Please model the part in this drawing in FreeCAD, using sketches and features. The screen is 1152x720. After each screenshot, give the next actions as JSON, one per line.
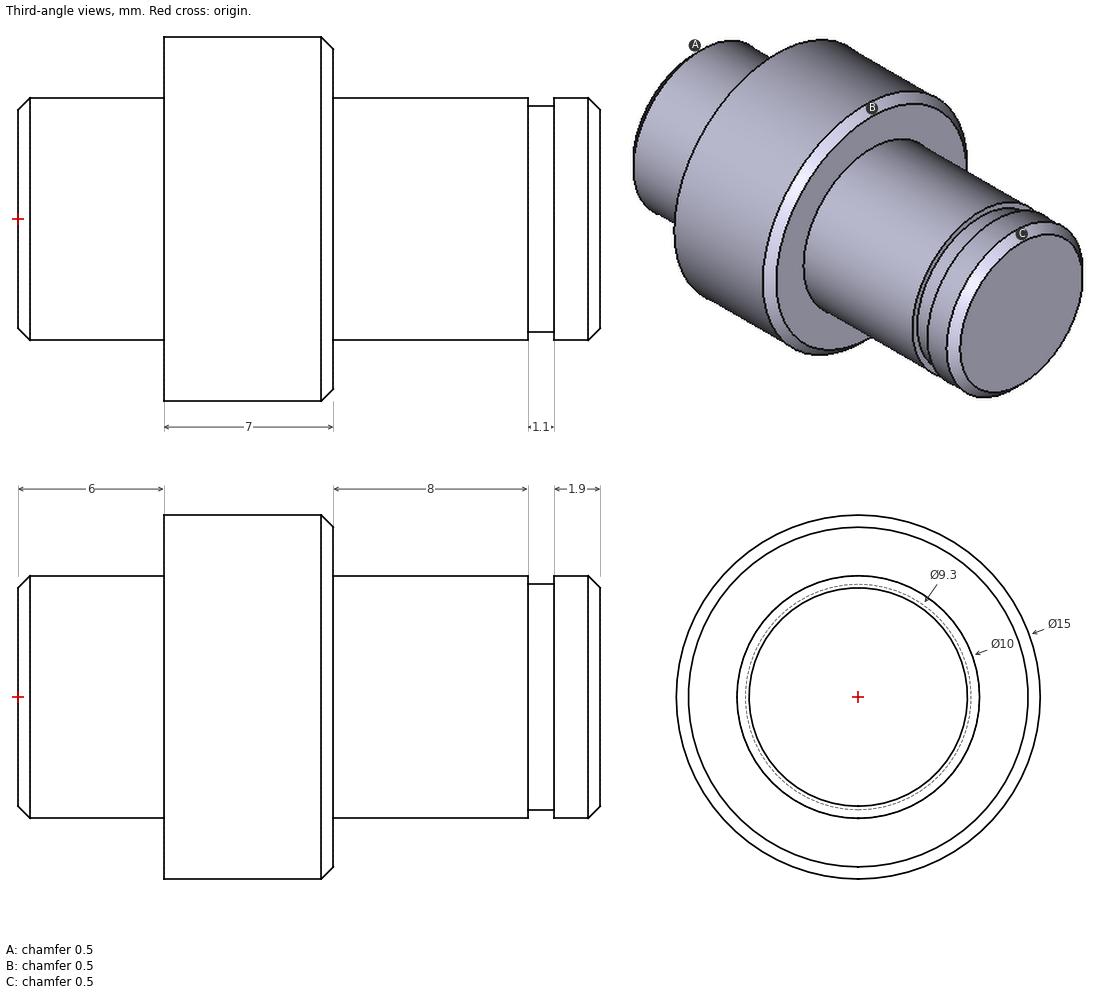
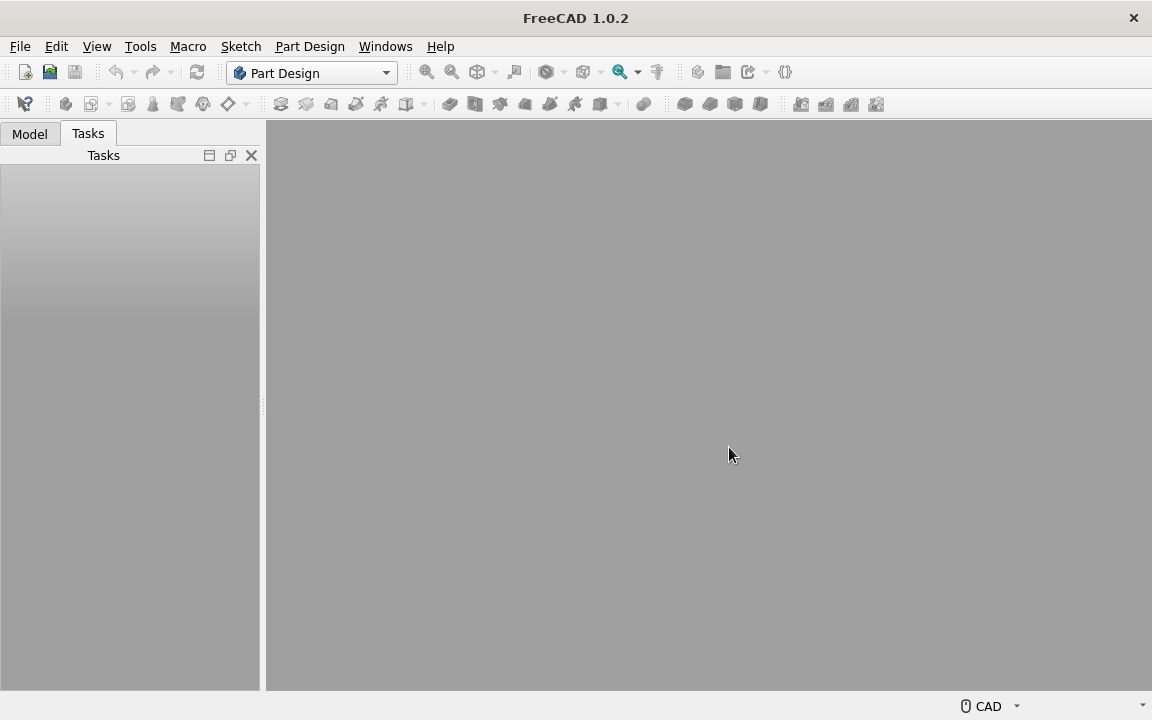
{"action": "left_click", "coordinate": [25, 72]}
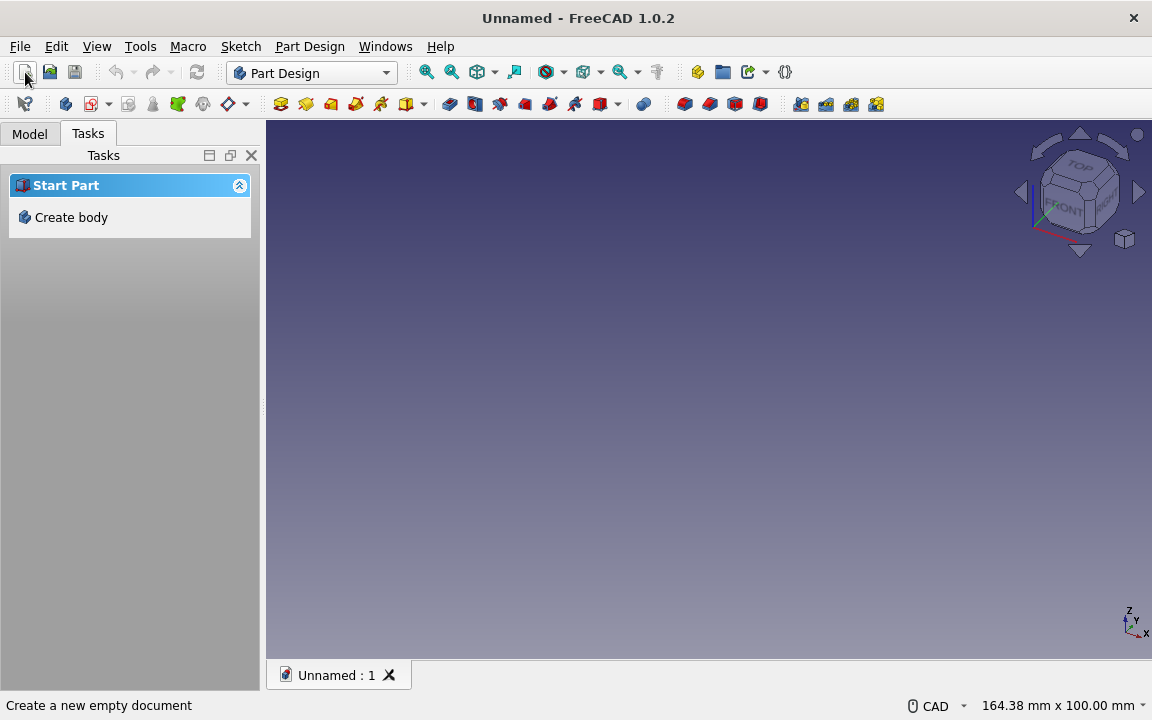
{"action": "left_click", "coordinate": [90, 104]}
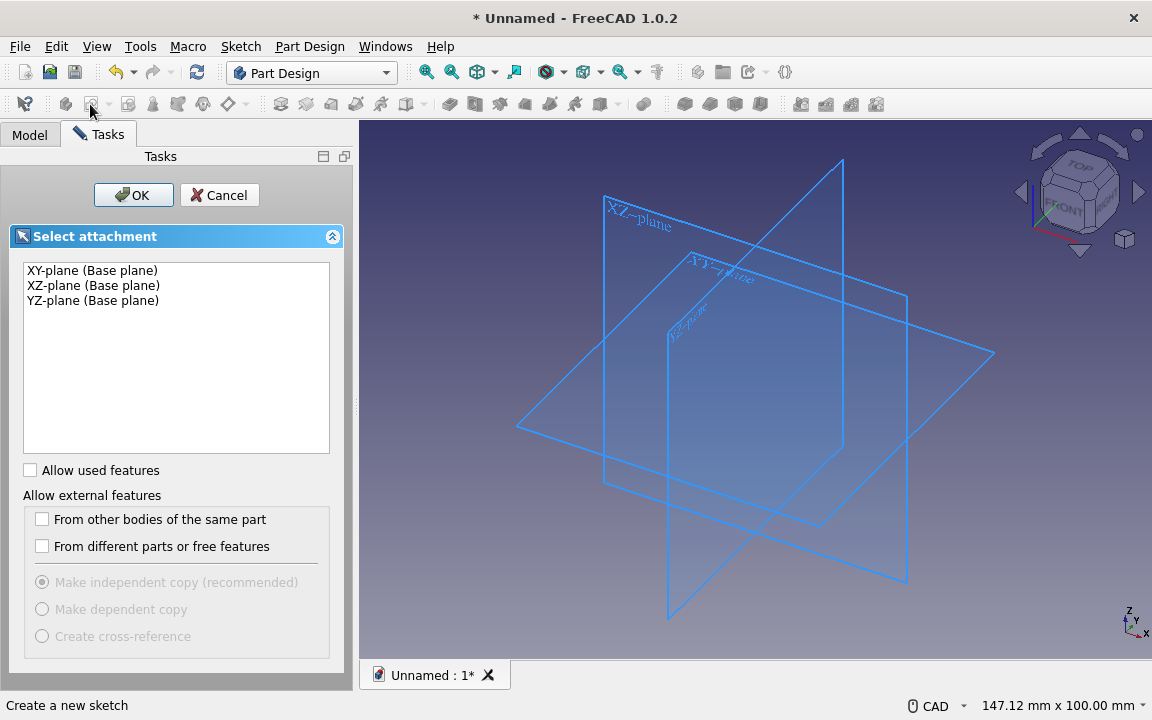
{"action": "left_click", "coordinate": [84, 300]}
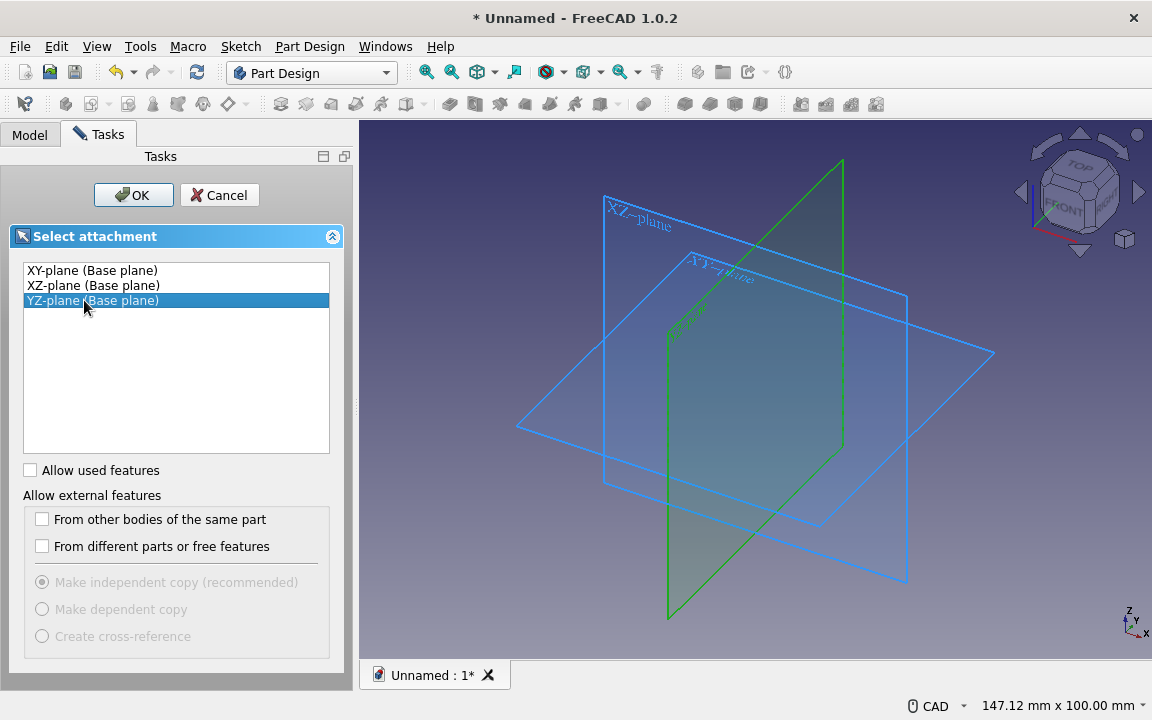
{"action": "left_click", "coordinate": [134, 195]}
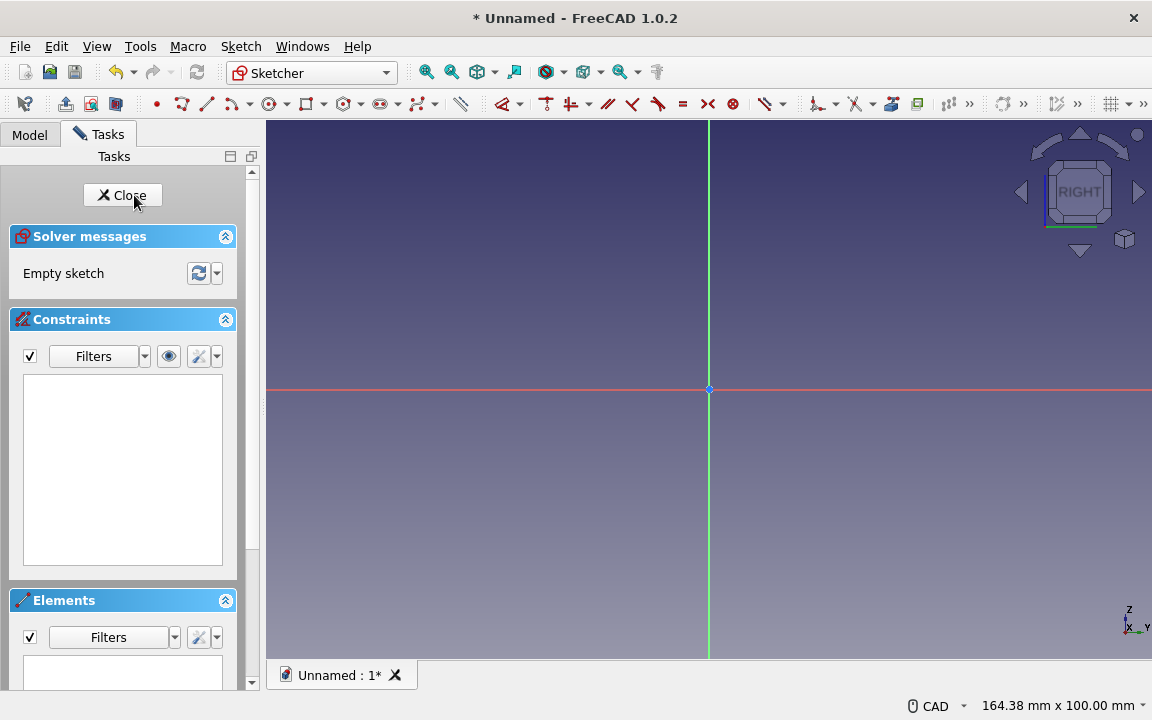
{"action": "scroll", "coordinate": [723, 390], "scroll_direction": "up", "scroll_amount": 9}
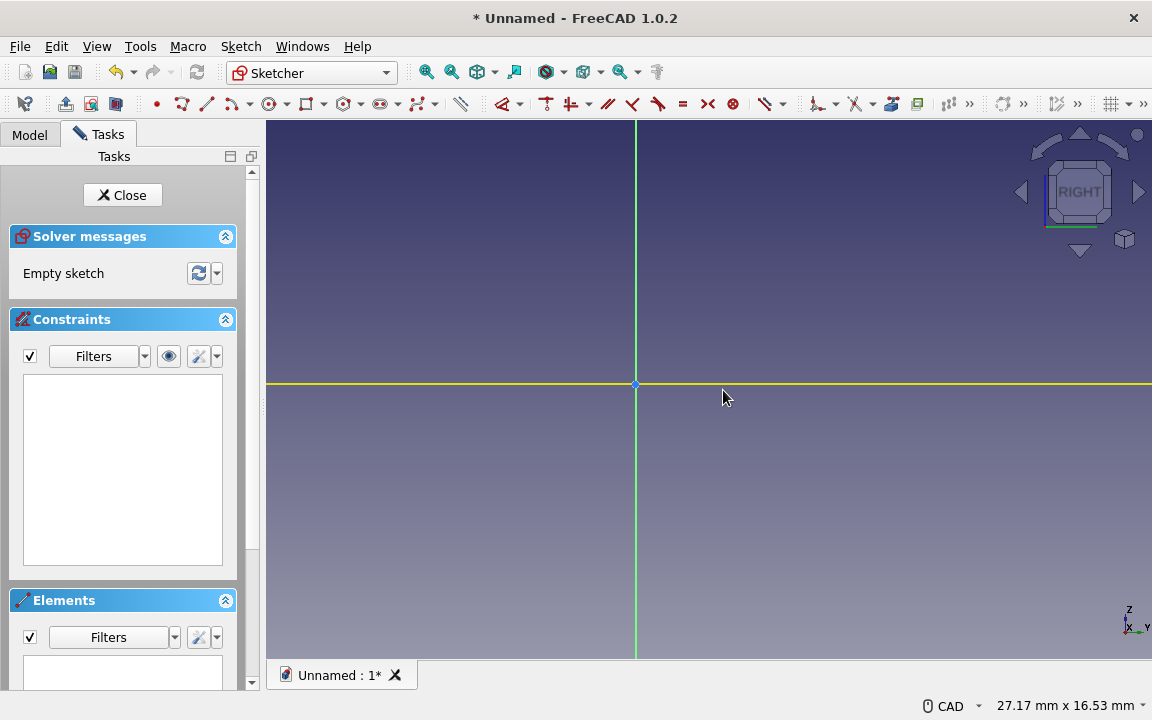
{"action": "key", "text": "g c"}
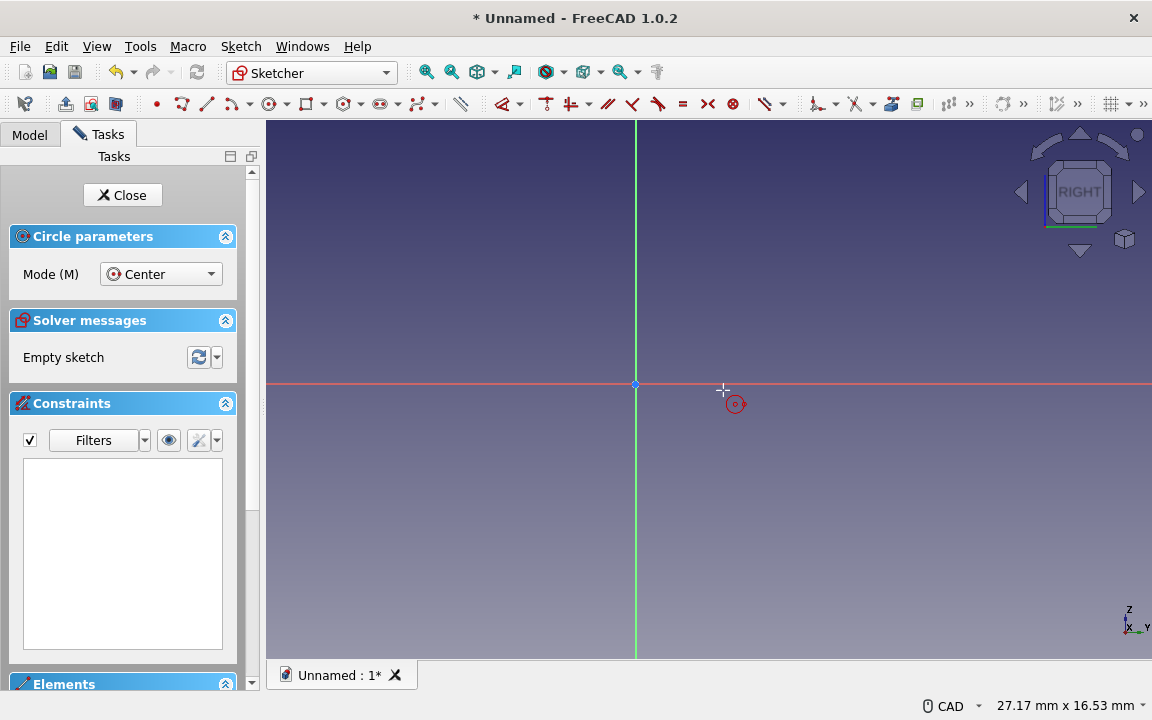
{"action": "left_click", "coordinate": [636, 384]}
{"action": "mouse_move", "coordinate": [751, 269]}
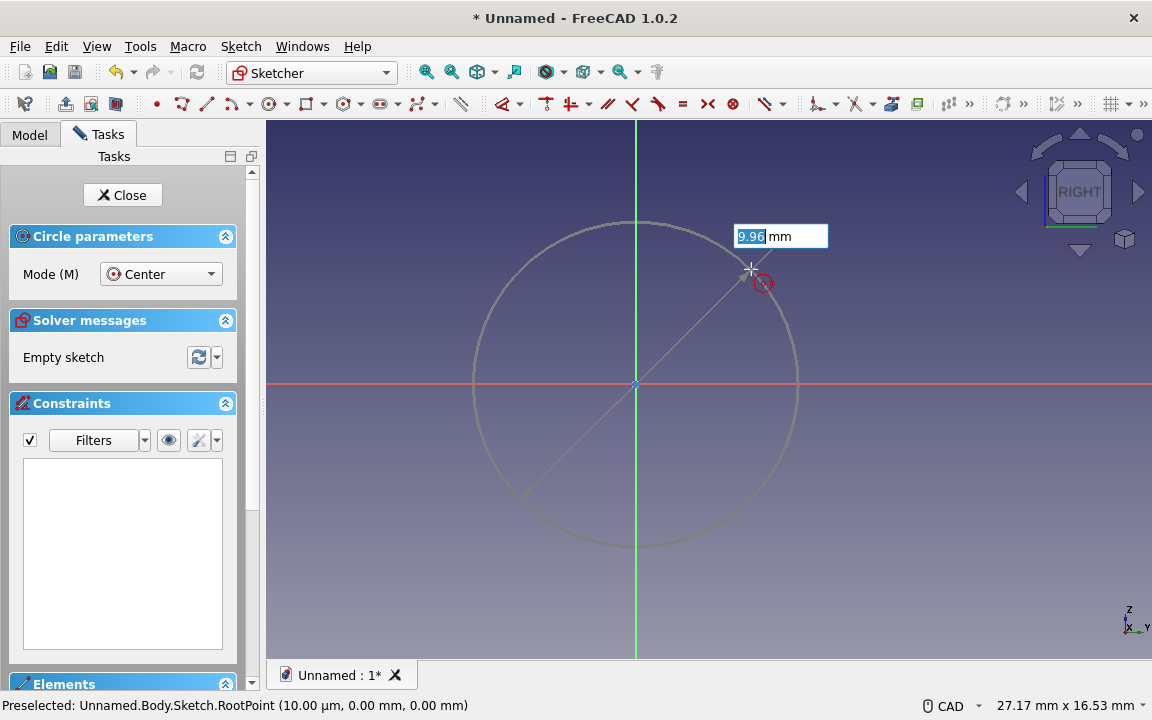
{"action": "type", "text": "10"}
{"action": "key", "text": "Return"}
{"action": "key", "text": "Escape"}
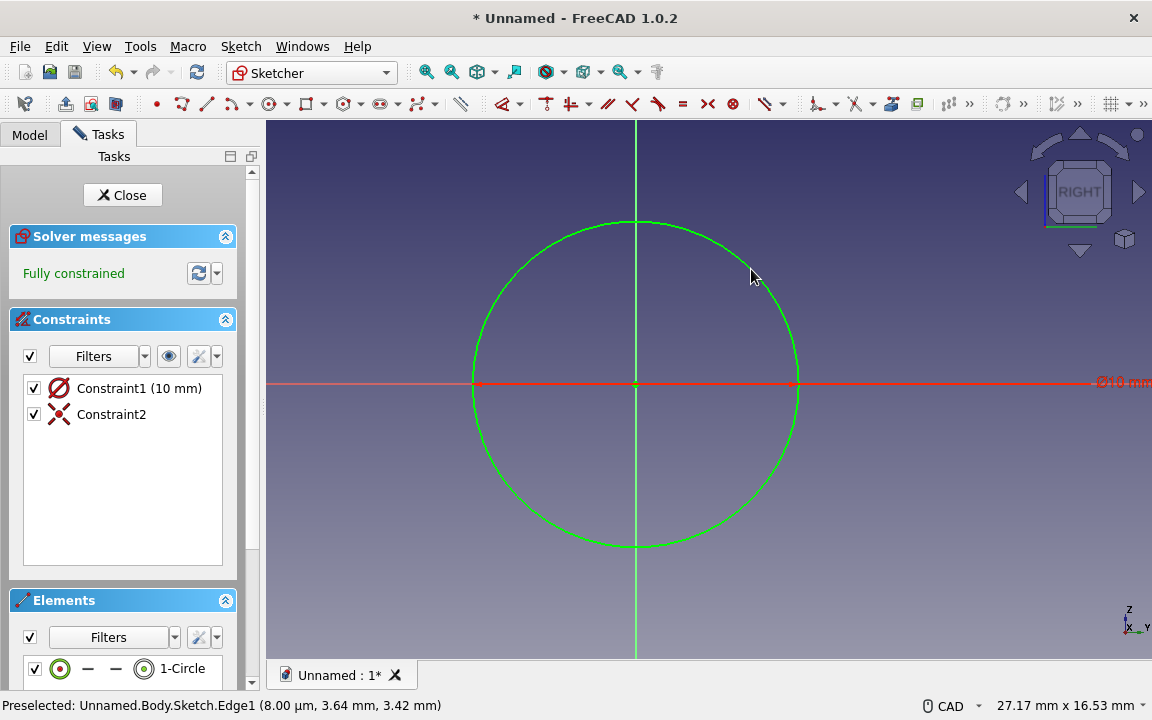
{"action": "left_click", "coordinate": [123, 195]}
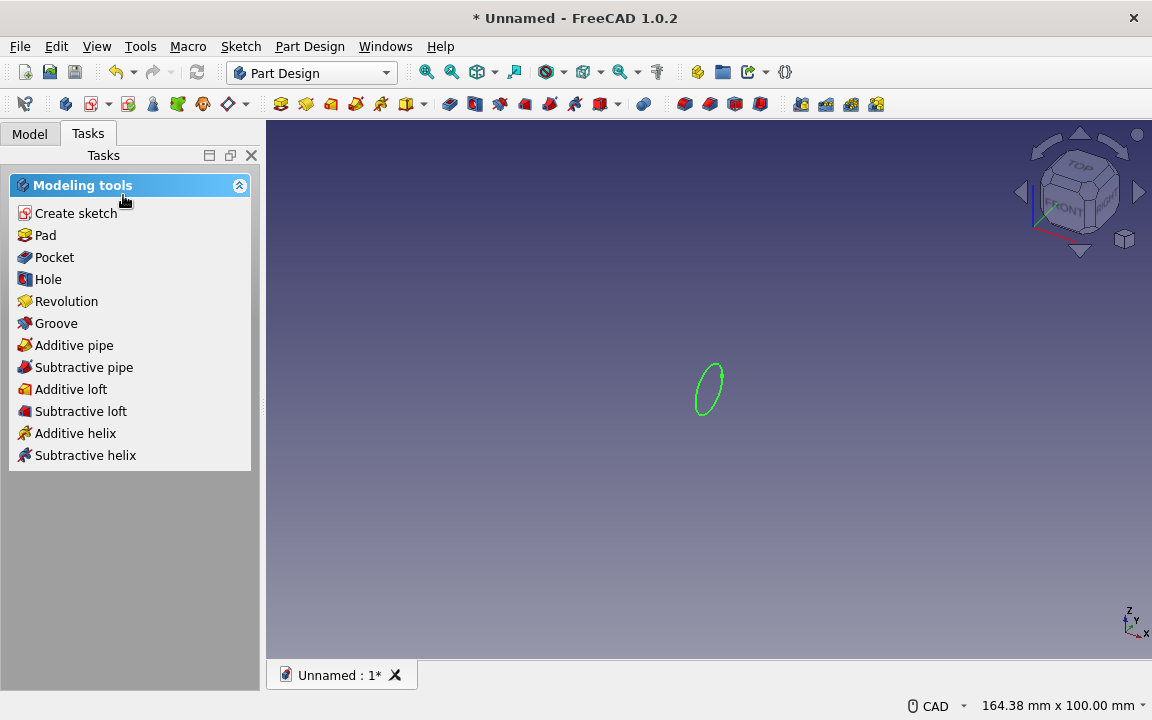
{"action": "left_click", "coordinate": [281, 104]}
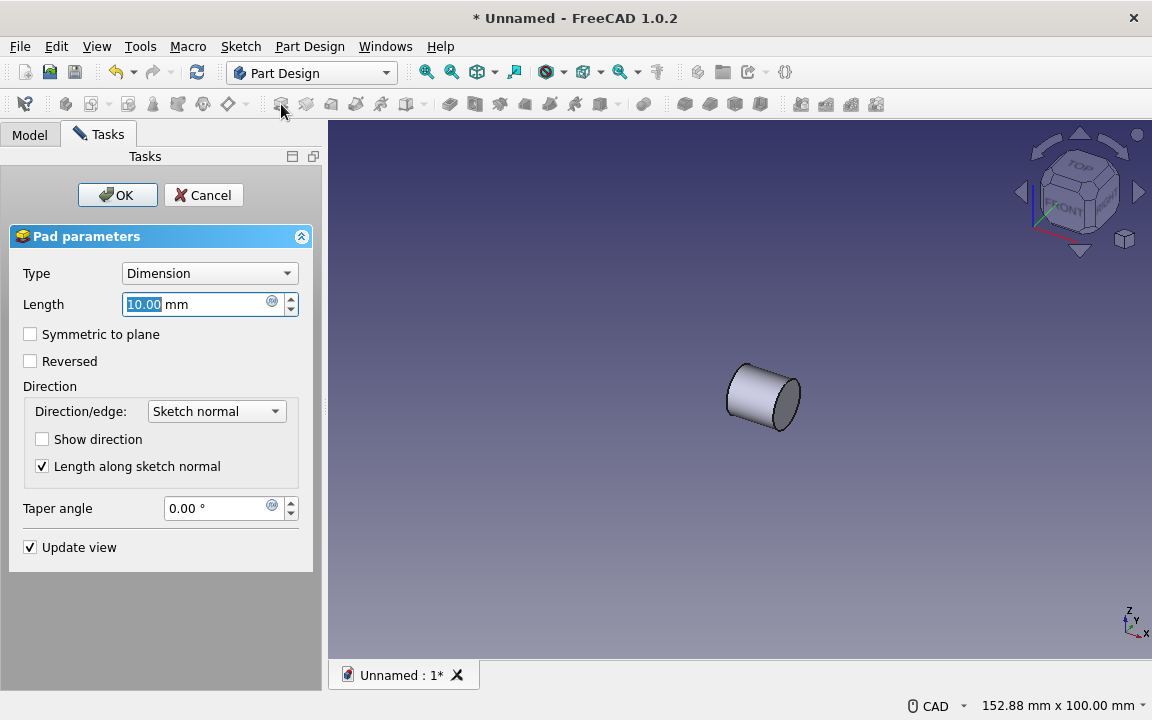
{"action": "type", "text": "6"}
{"action": "key", "text": "Tab"}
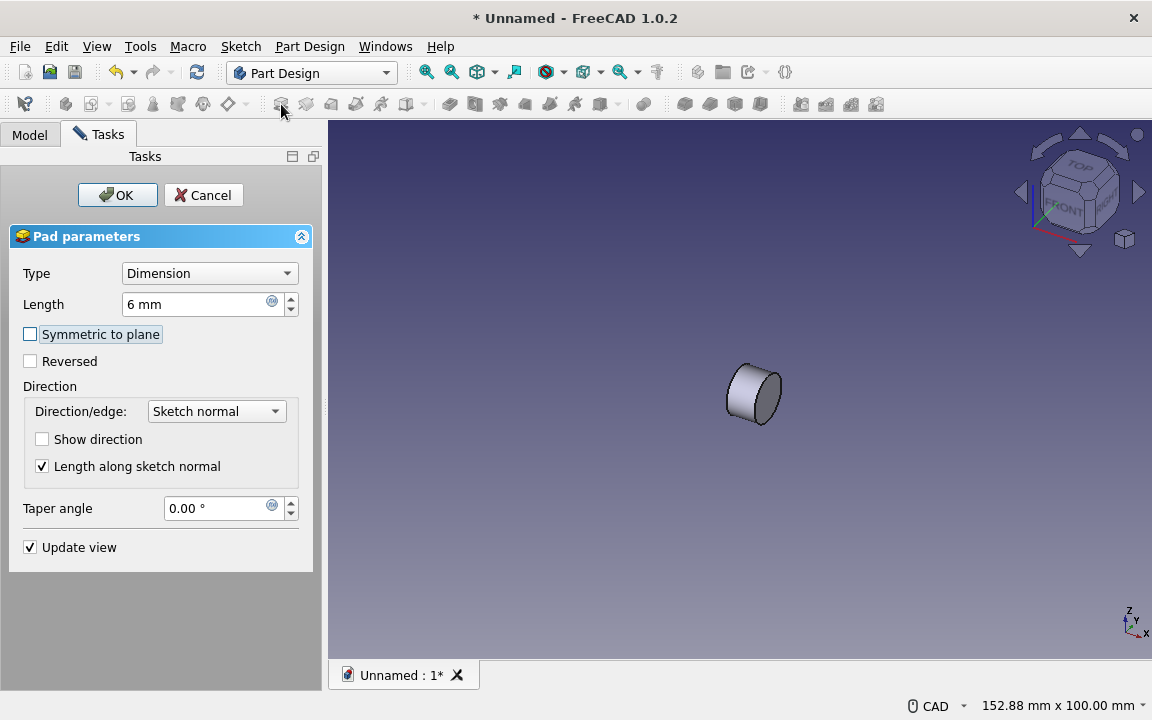
{"action": "left_click", "coordinate": [118, 195]}